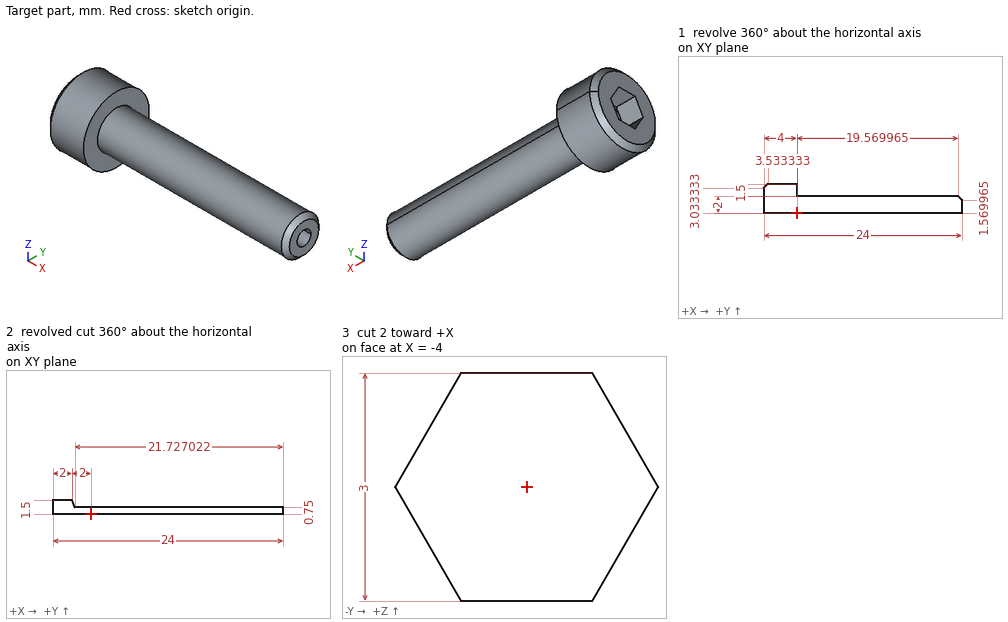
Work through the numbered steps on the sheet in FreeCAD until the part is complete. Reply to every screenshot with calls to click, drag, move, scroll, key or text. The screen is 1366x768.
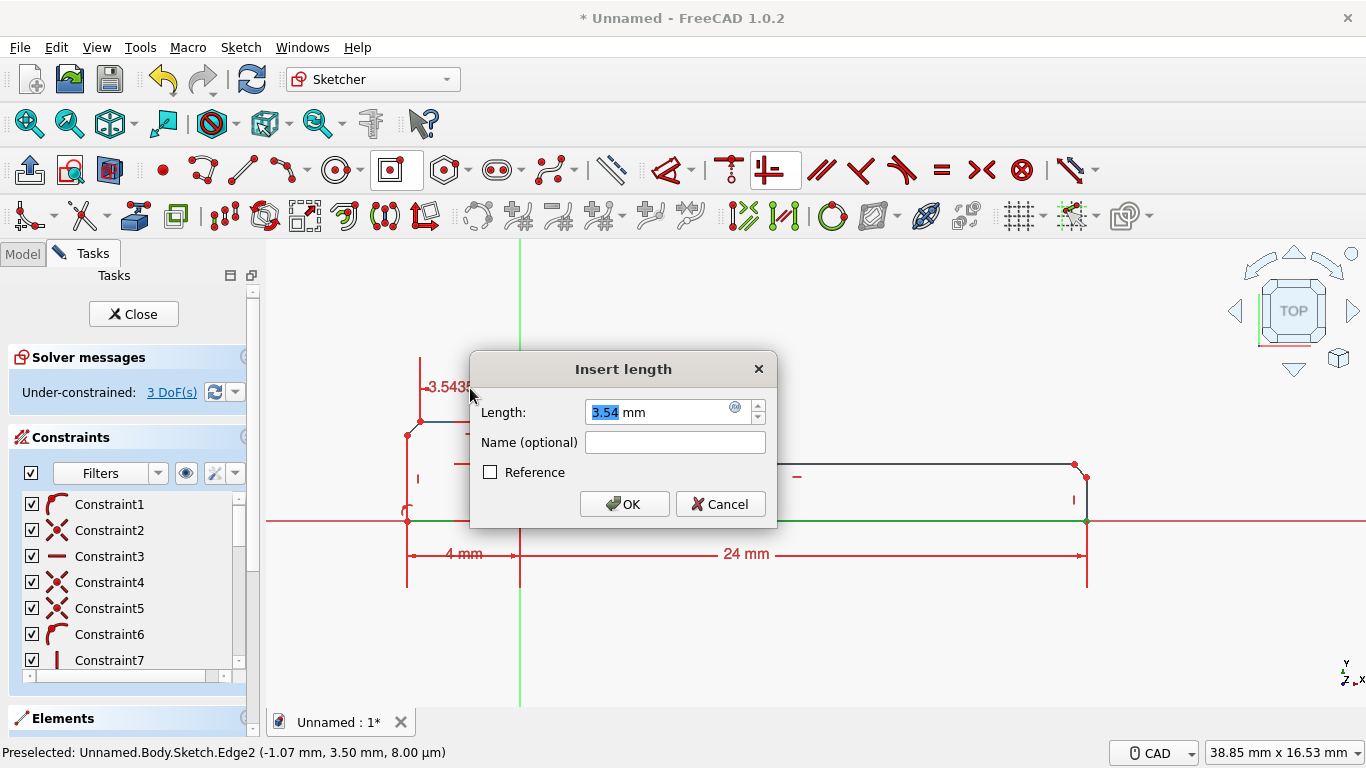
text(3.533333)
key(Return)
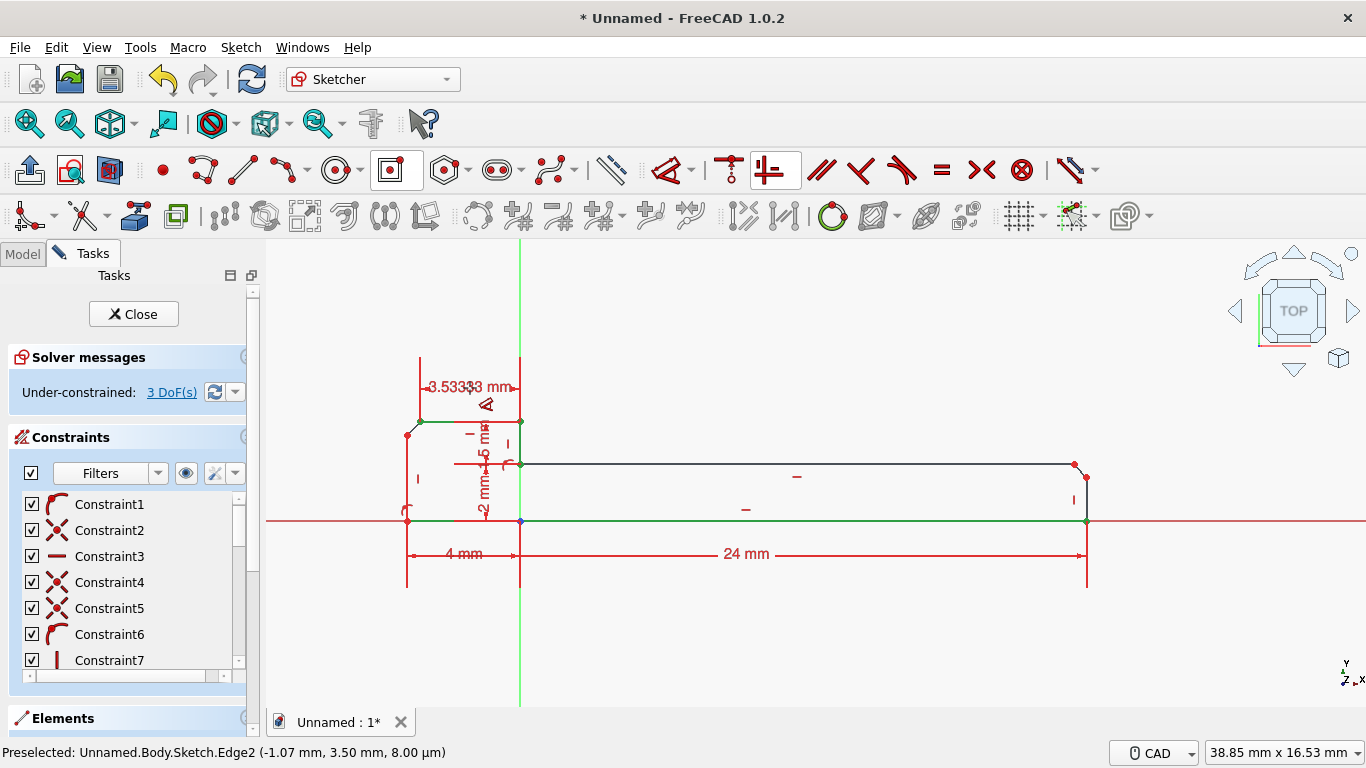
click(407, 462)
click(373, 479)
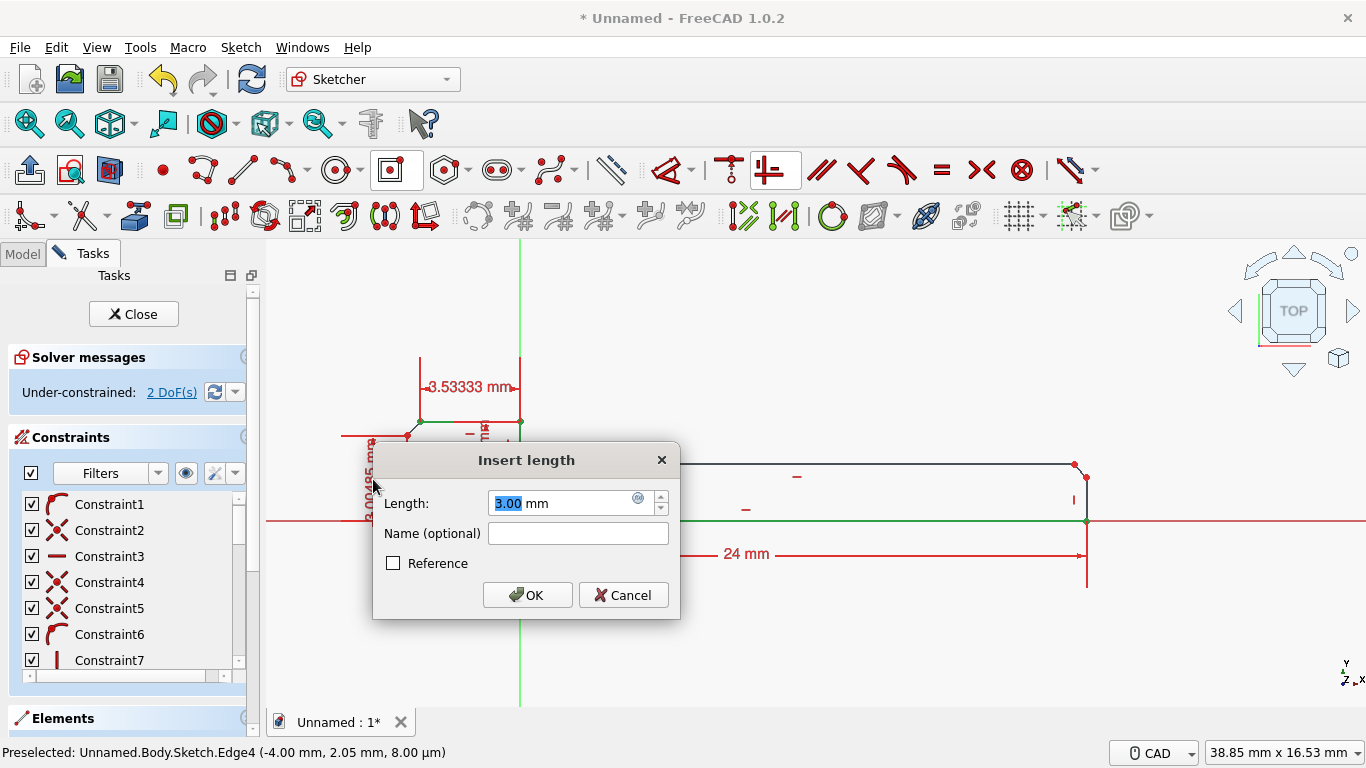
text(3.033333)
key(Return)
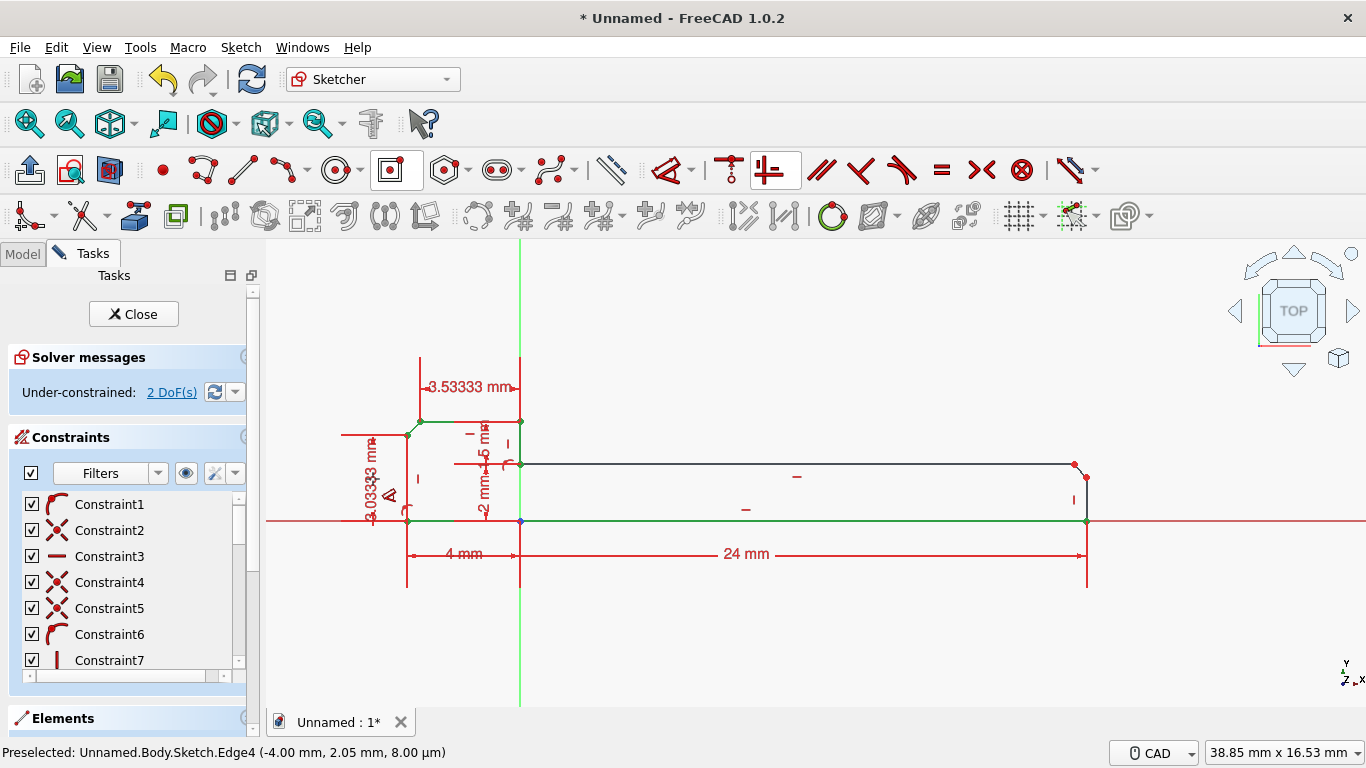
click(1087, 508)
click(1121, 500)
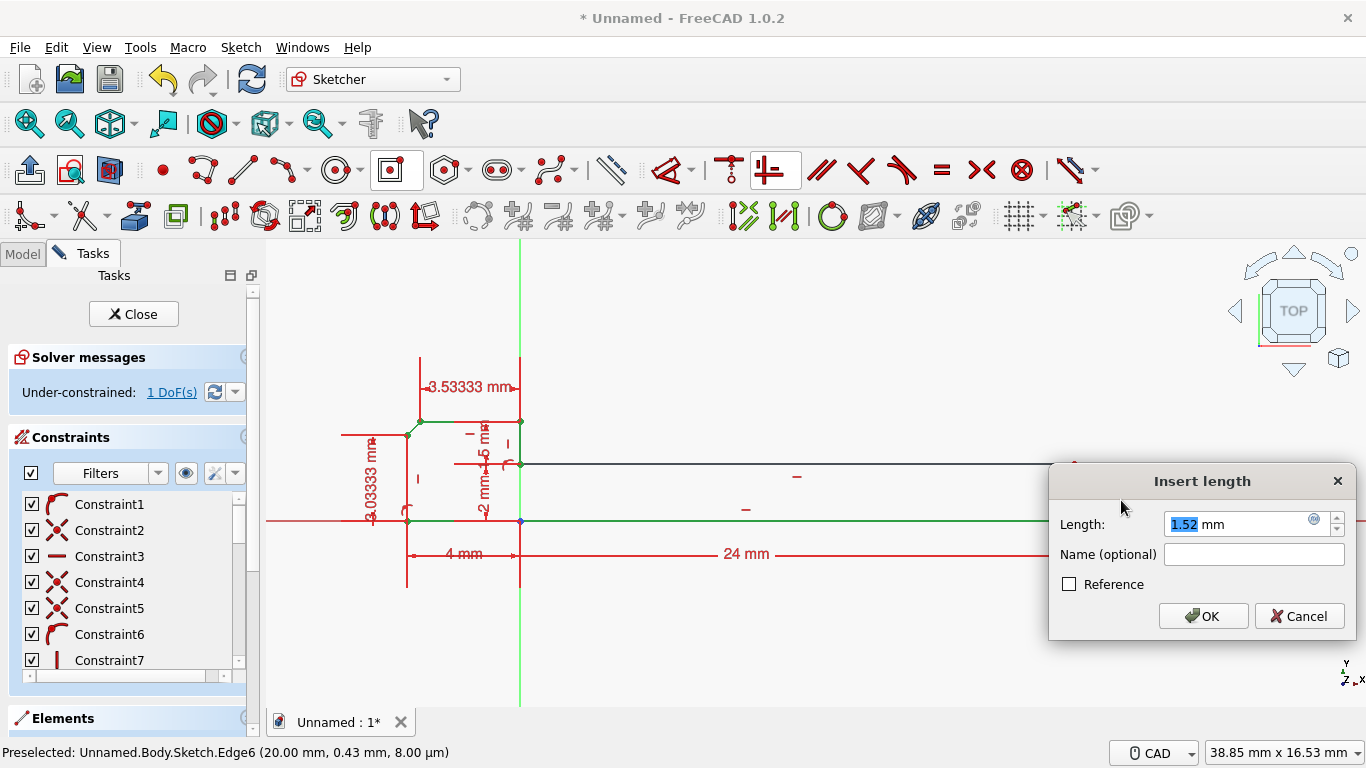
text(1.569965)
key(Return)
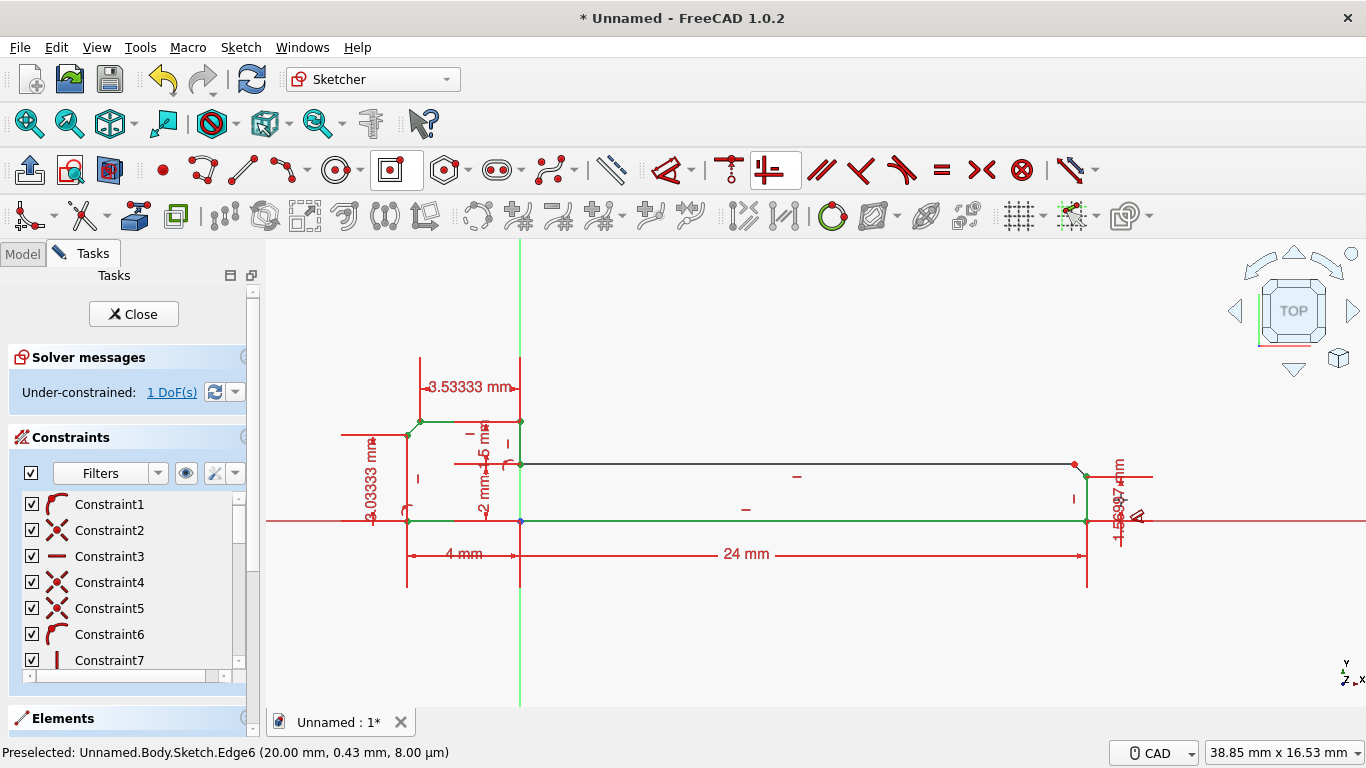
click(908, 464)
click(797, 430)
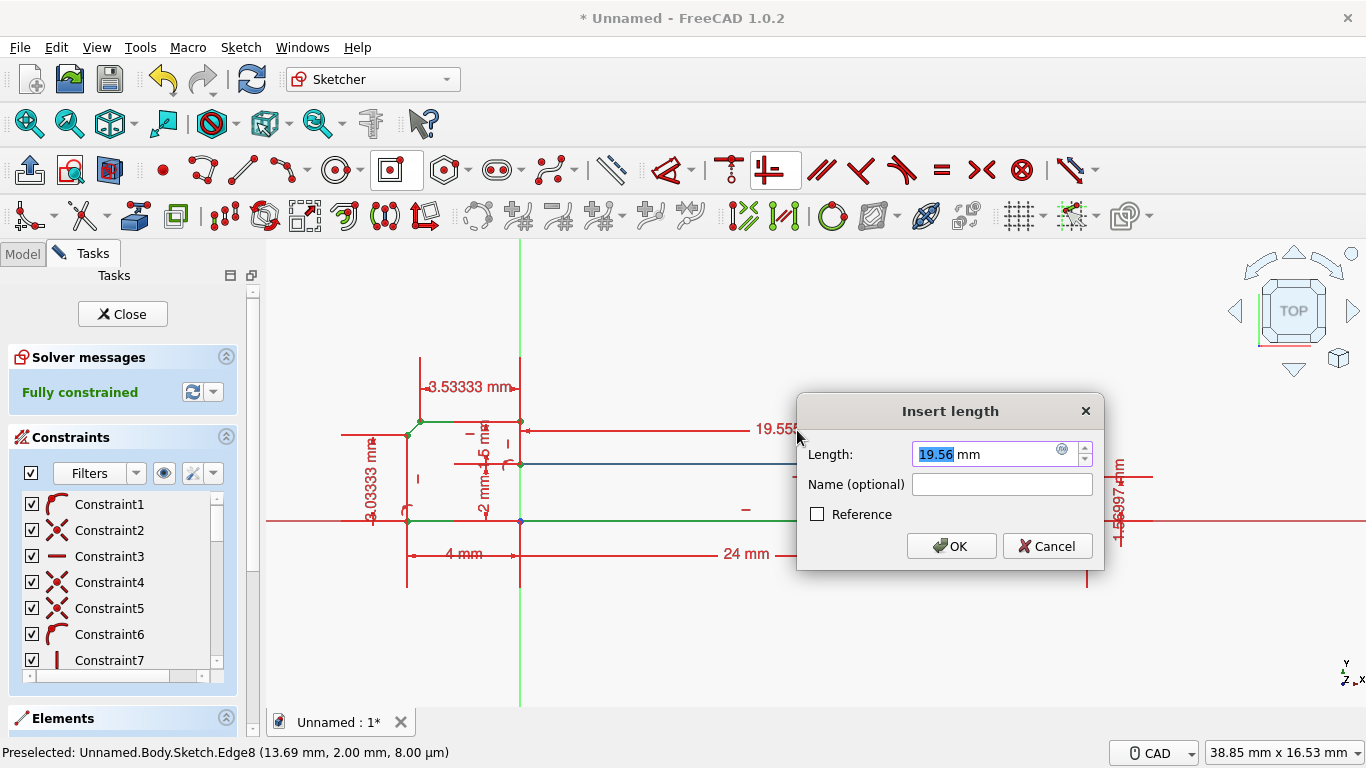
text(19.569965)
key(Return)
key(Escape)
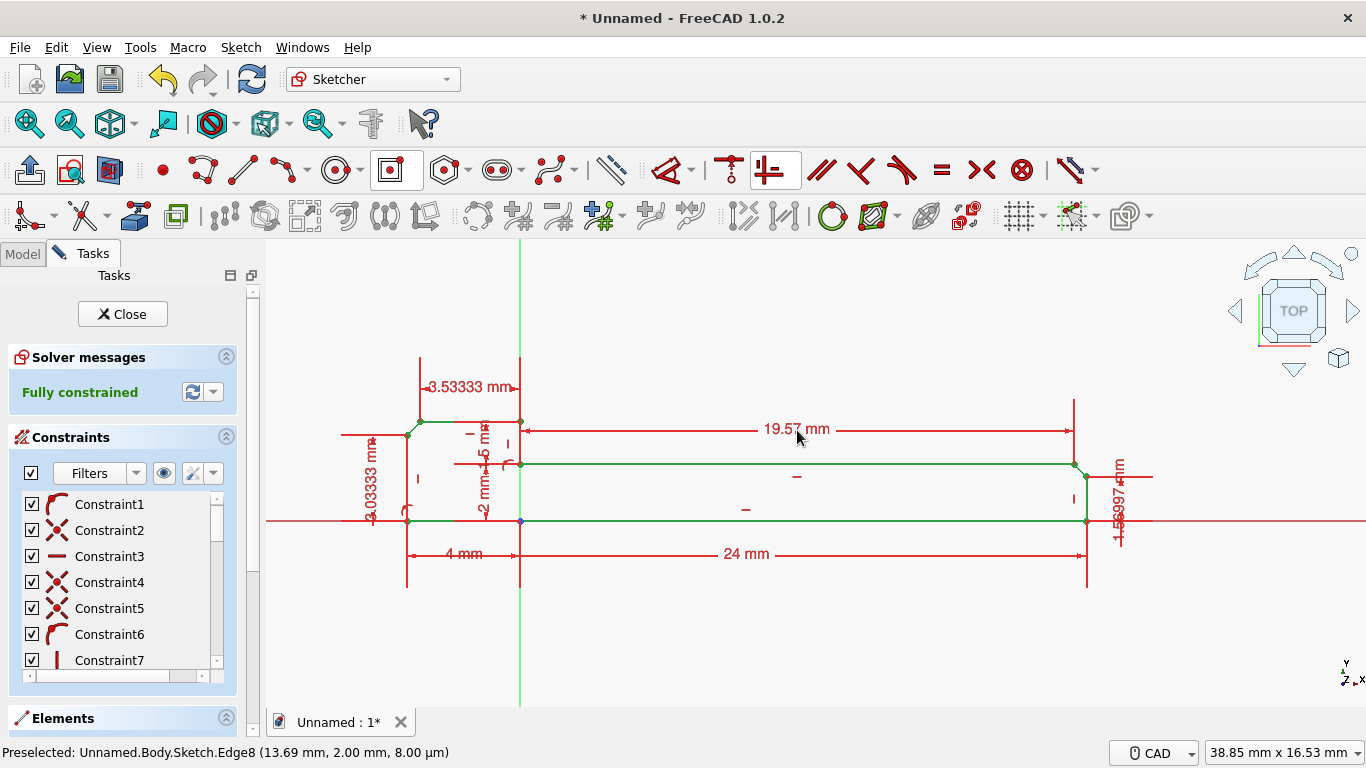
click(123, 314)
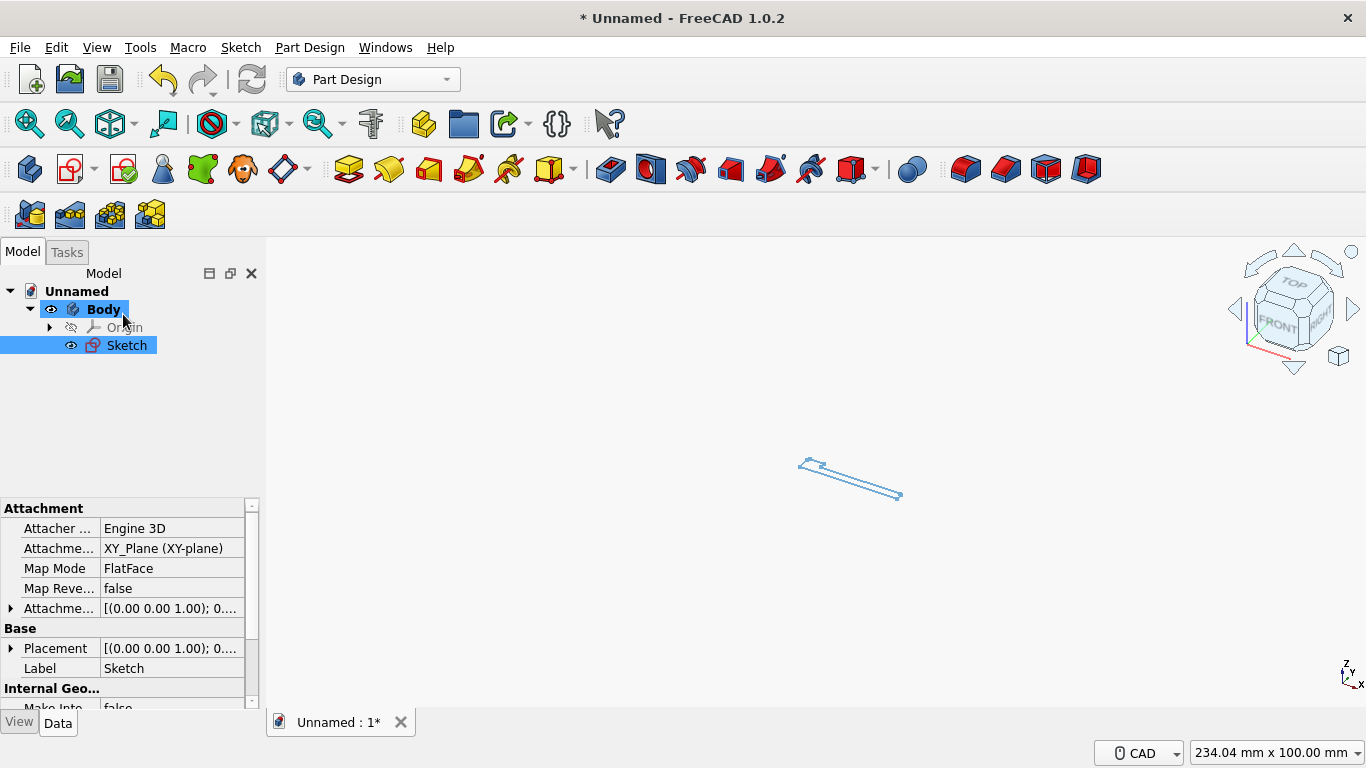
click(390, 170)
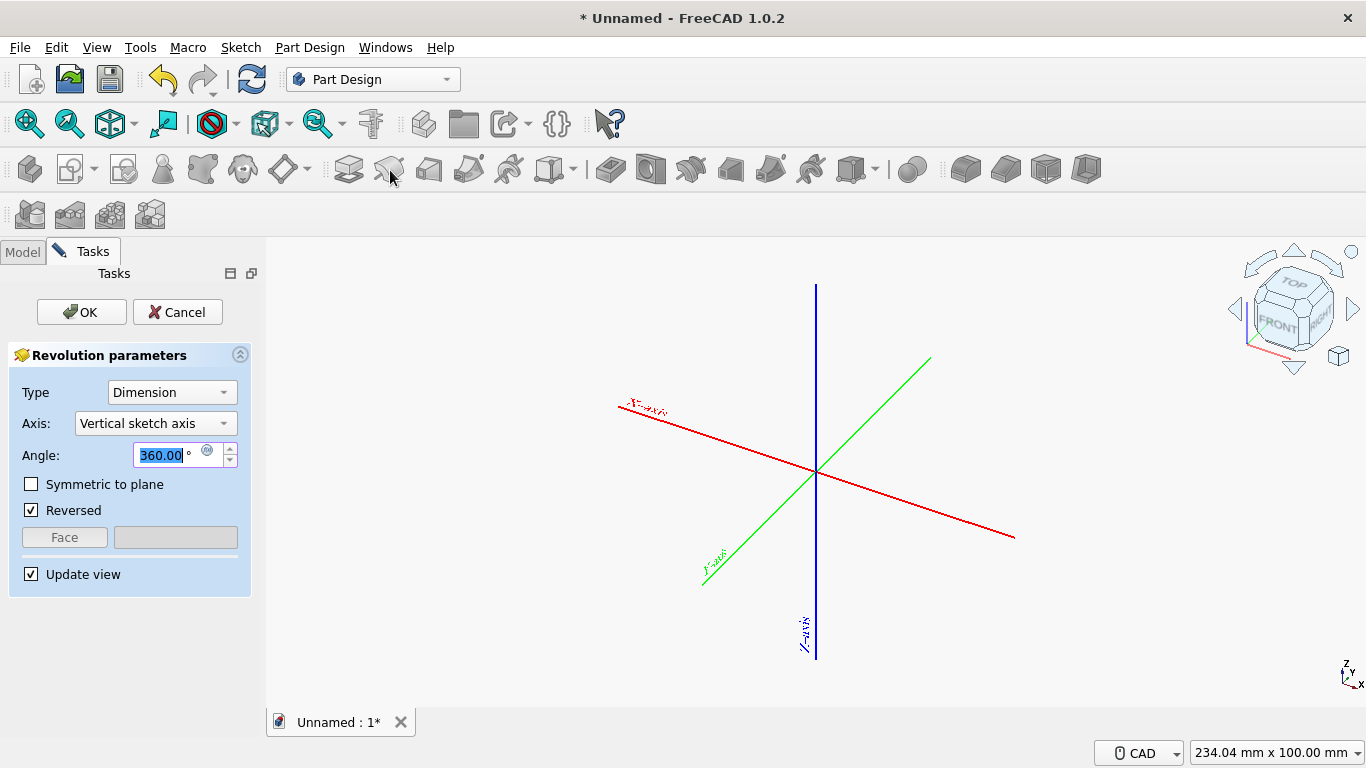
click(156, 424)